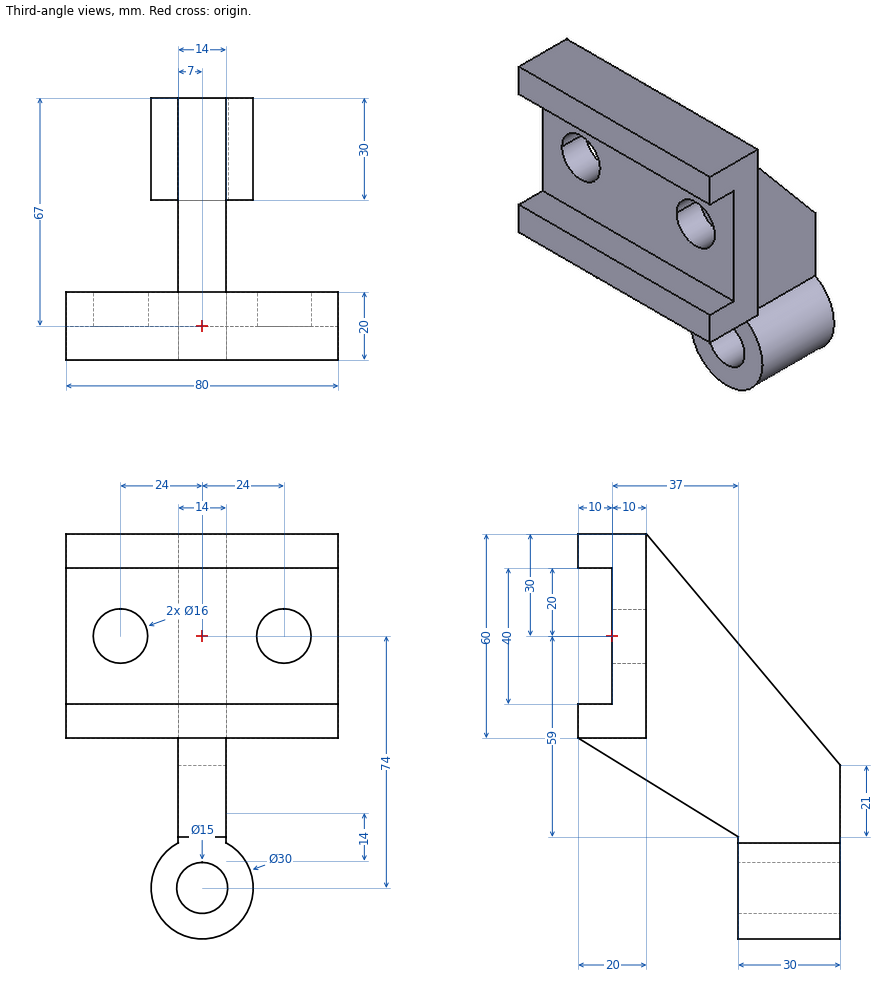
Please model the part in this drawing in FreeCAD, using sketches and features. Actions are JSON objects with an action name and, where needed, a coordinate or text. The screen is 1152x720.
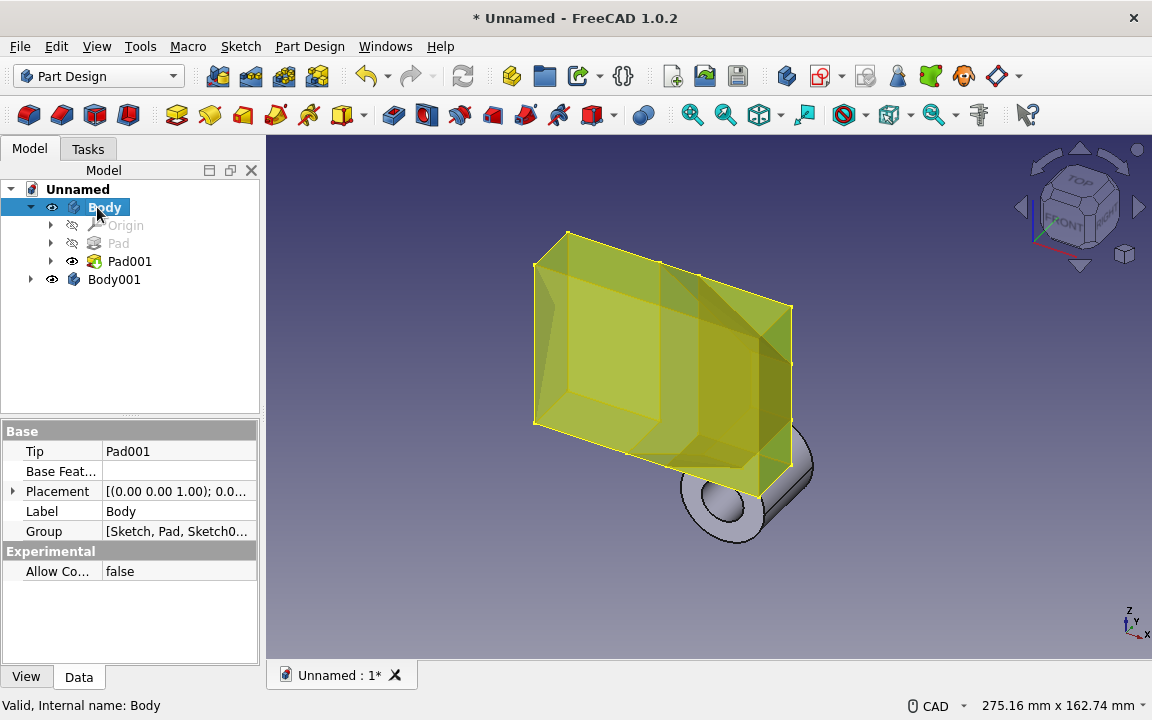
{"action": "left_click", "coordinate": [148, 571]}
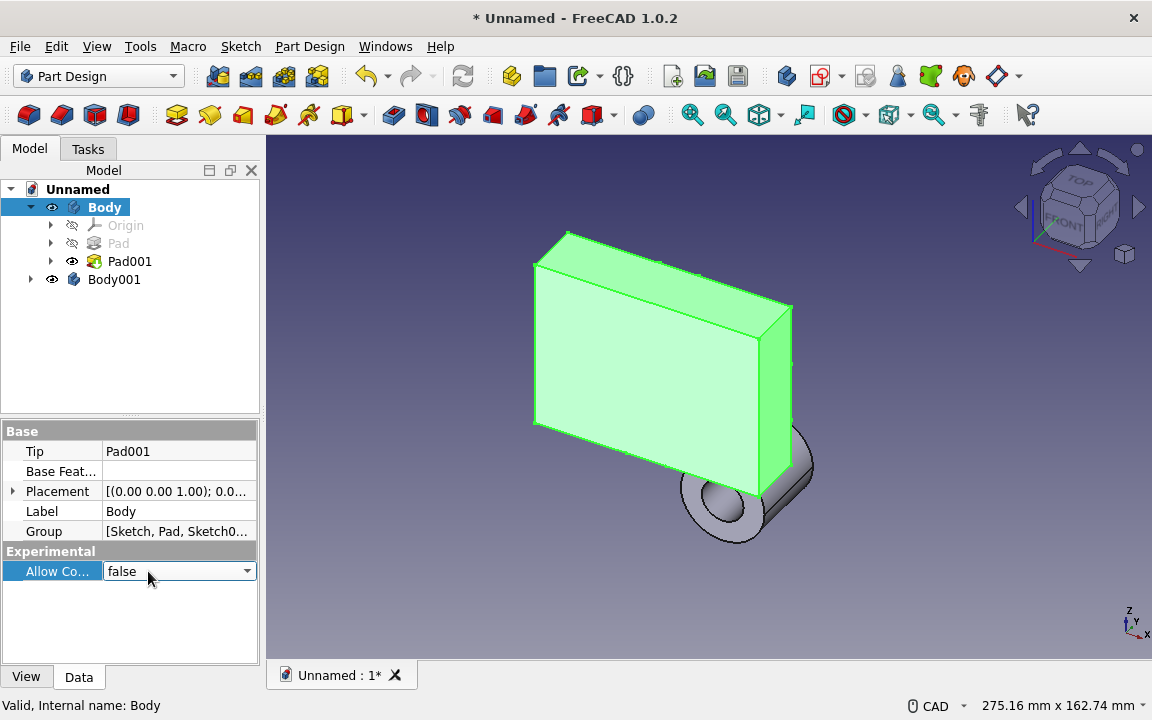
{"action": "left_click", "coordinate": [148, 571]}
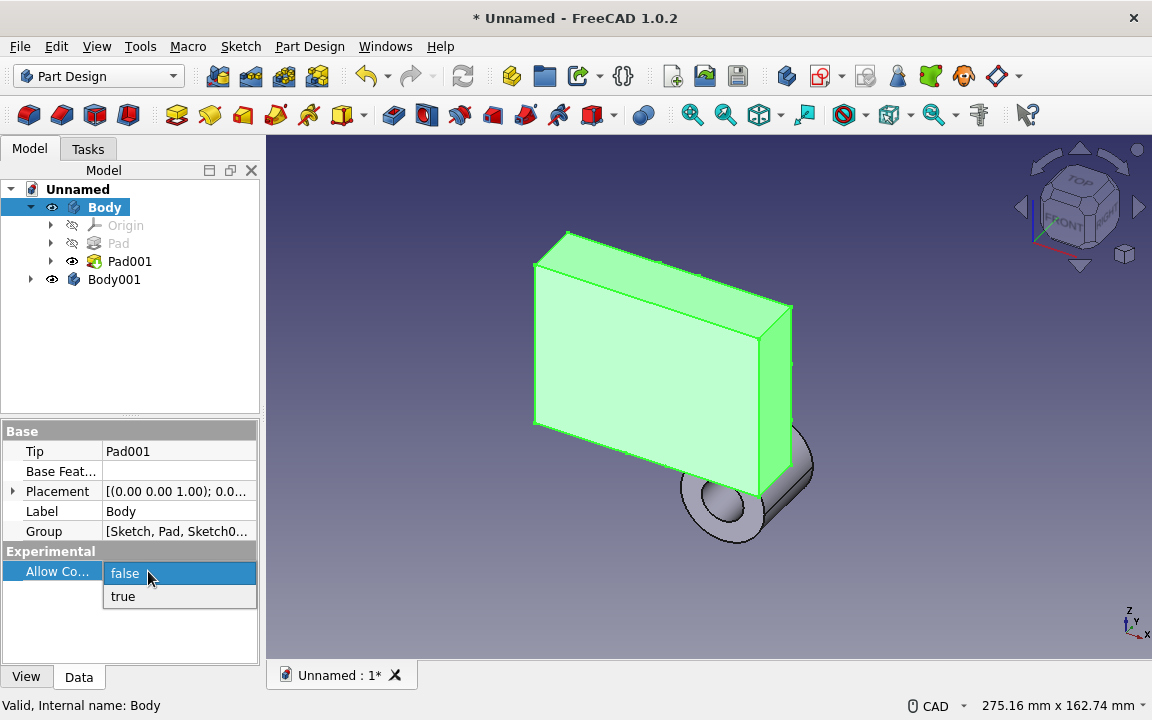
{"action": "left_click", "coordinate": [178, 596]}
{"action": "key", "text": "Return"}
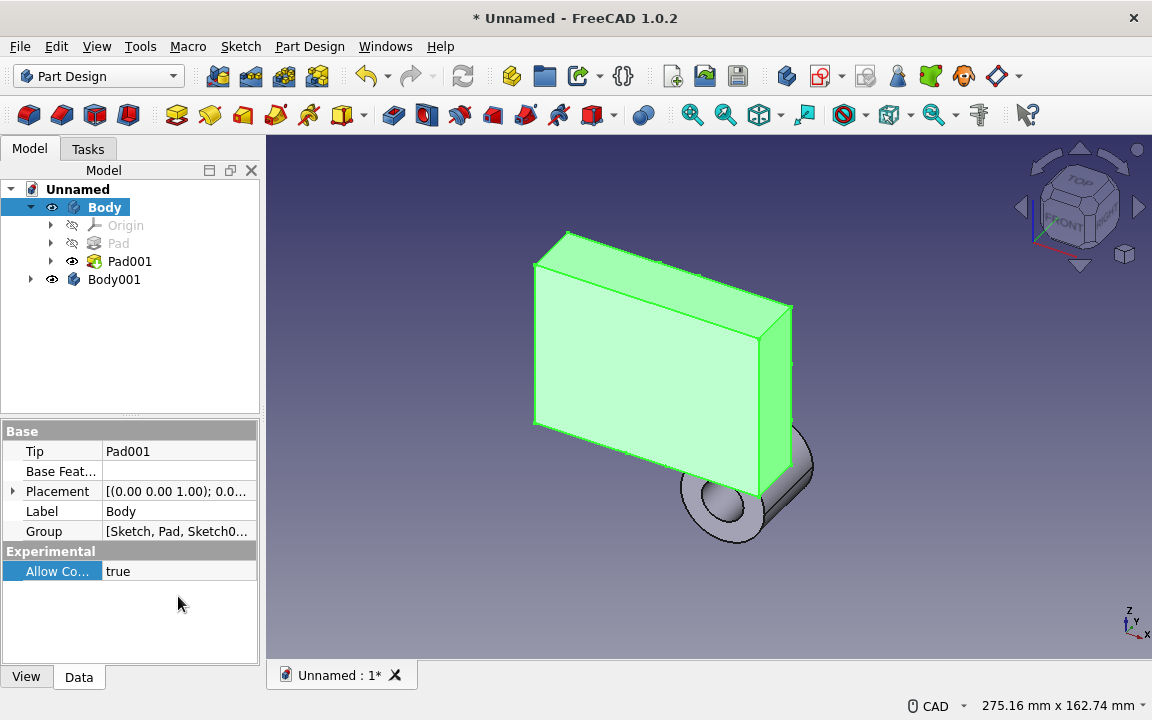
{"action": "left_click", "coordinate": [97, 279]}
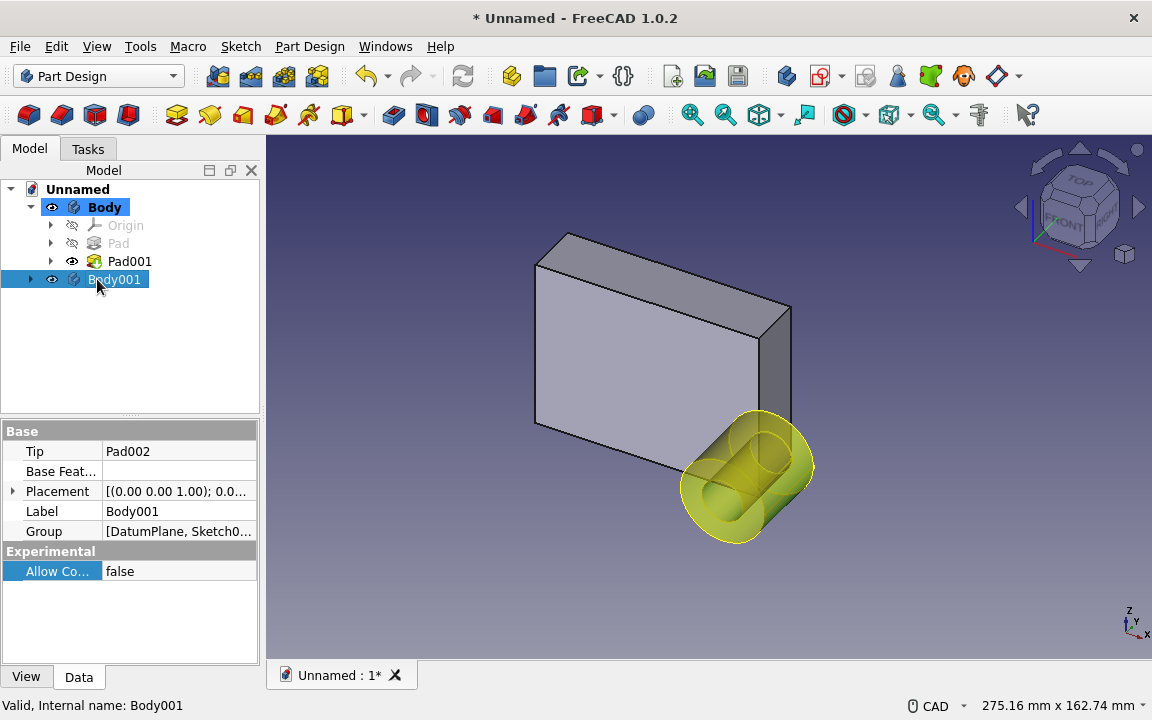
{"action": "left_click", "coordinate": [644, 116]}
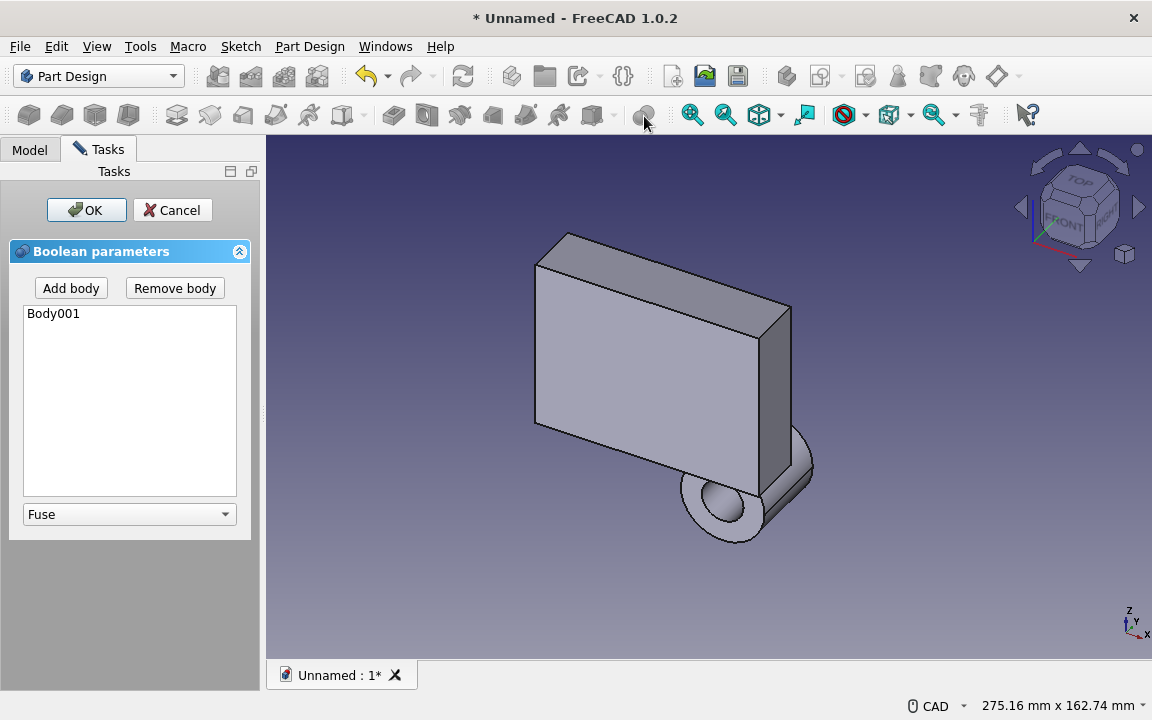
{"action": "left_click", "coordinate": [87, 210]}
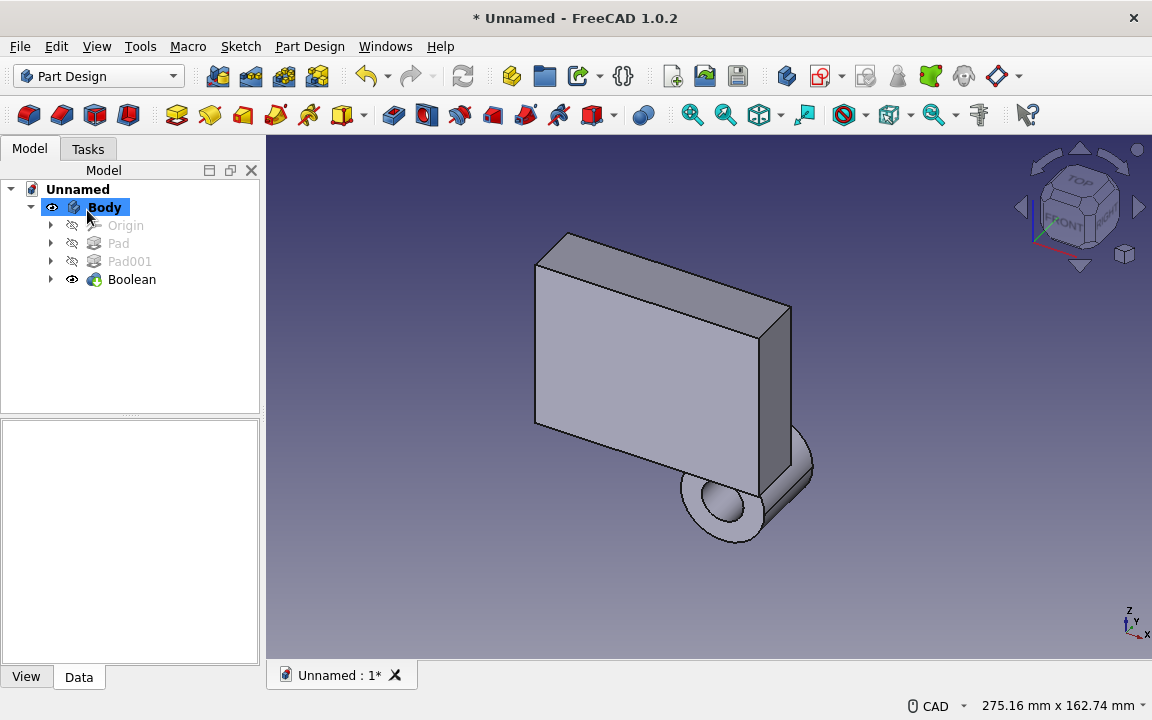
{"action": "left_click", "coordinate": [51, 225]}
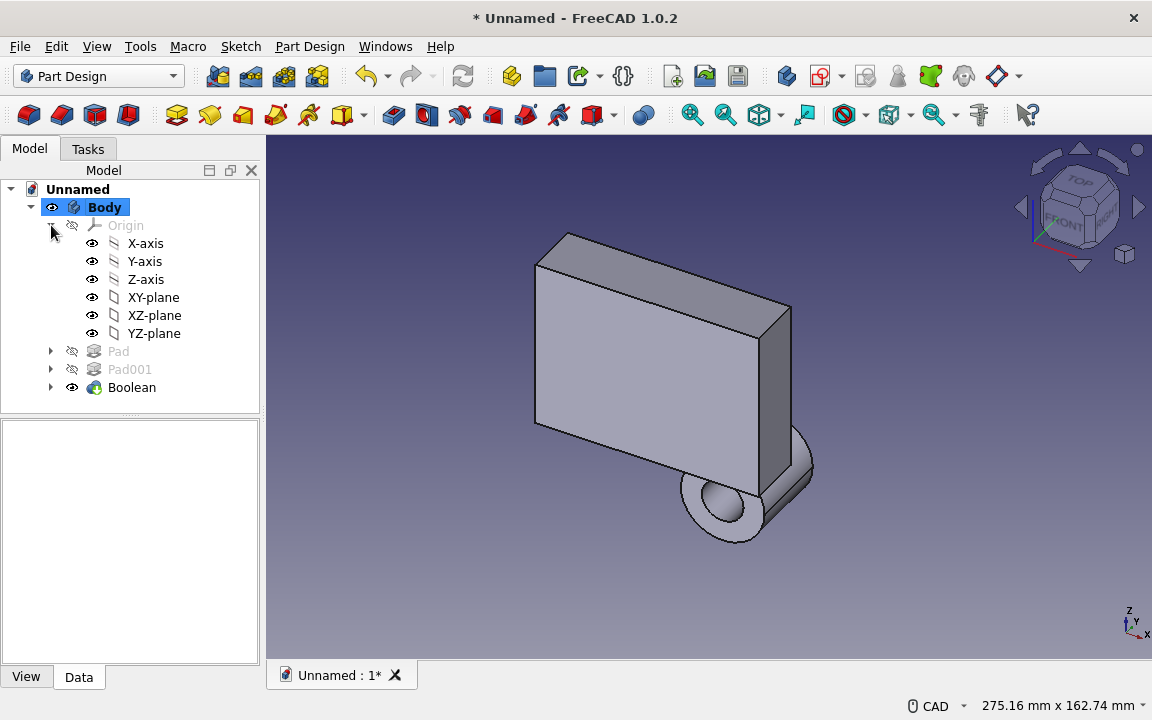
{"action": "left_click", "coordinate": [137, 297]}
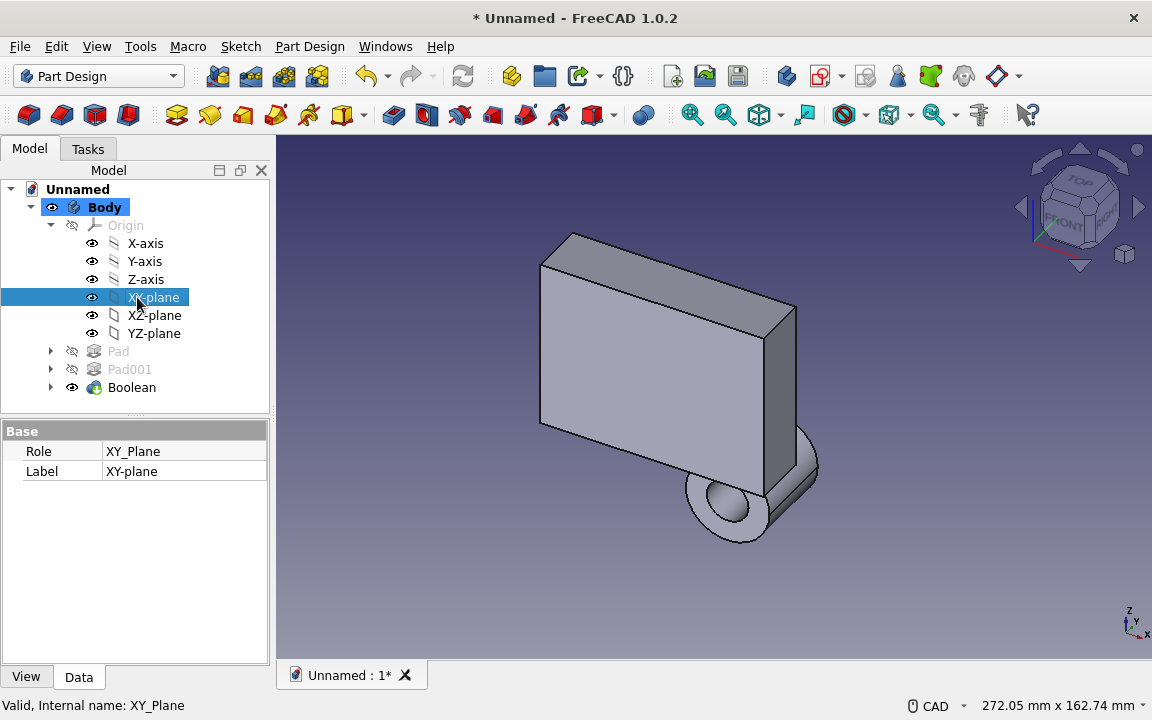
{"action": "left_click", "coordinate": [996, 76]}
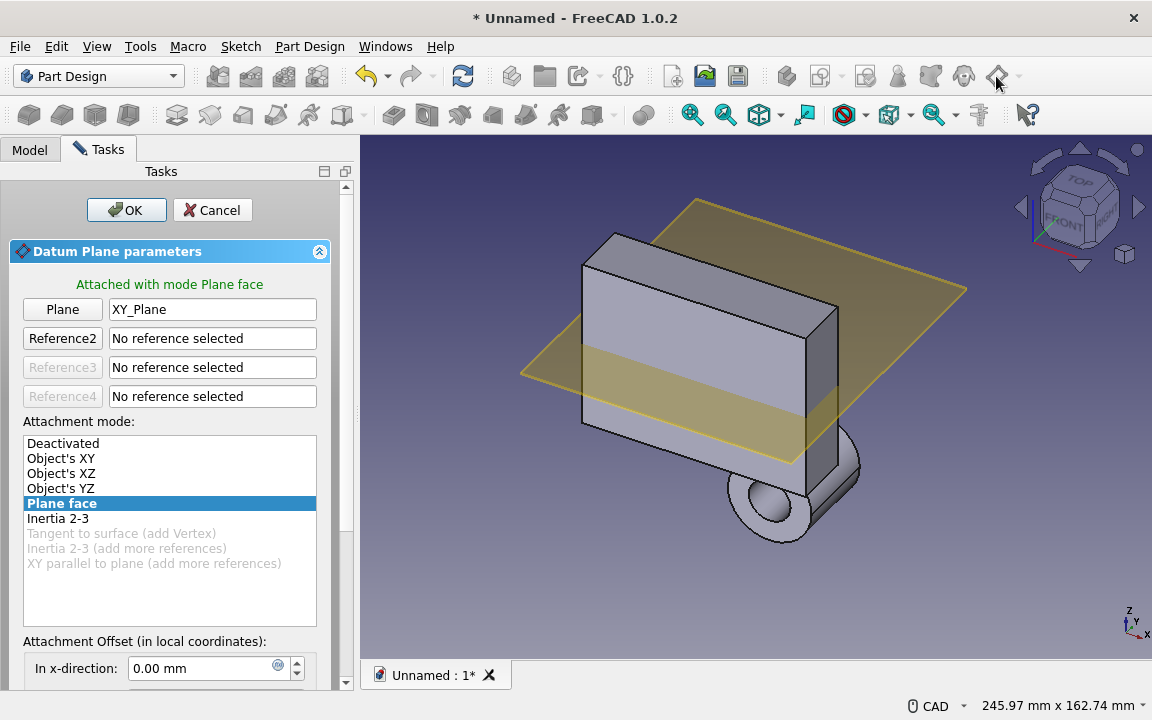
{"action": "scroll", "coordinate": [346, 436], "scroll_direction": "down", "scroll_amount": 2}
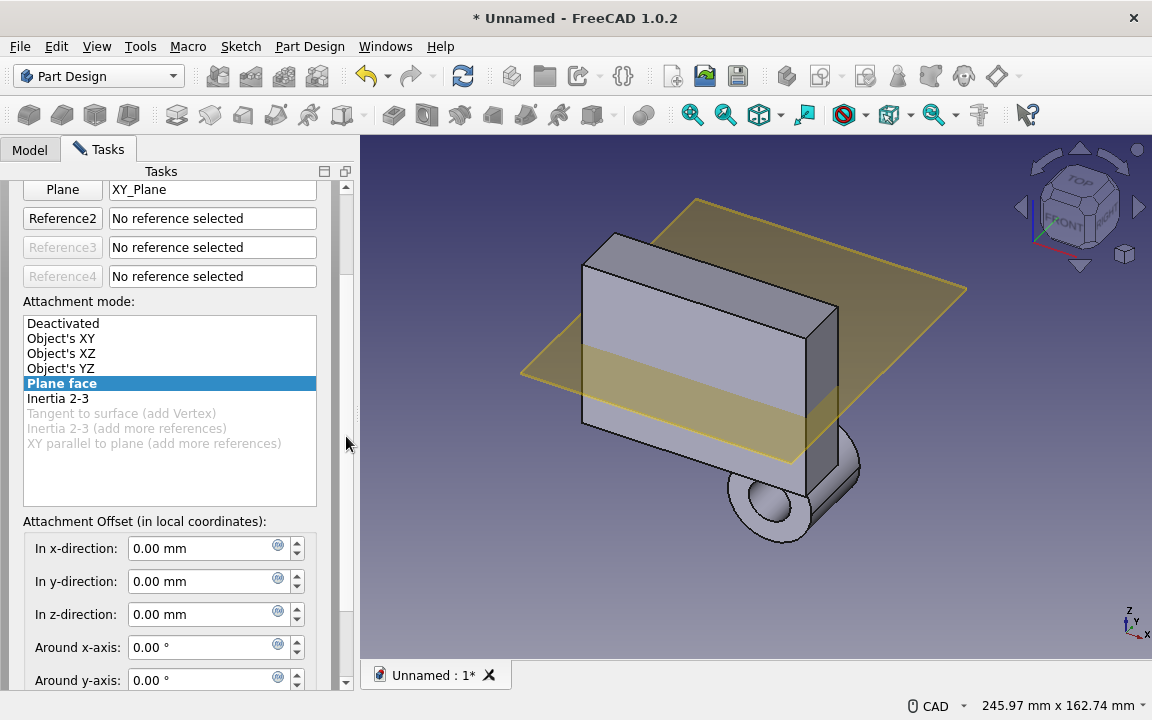
{"action": "triple_click", "coordinate": [210, 614]}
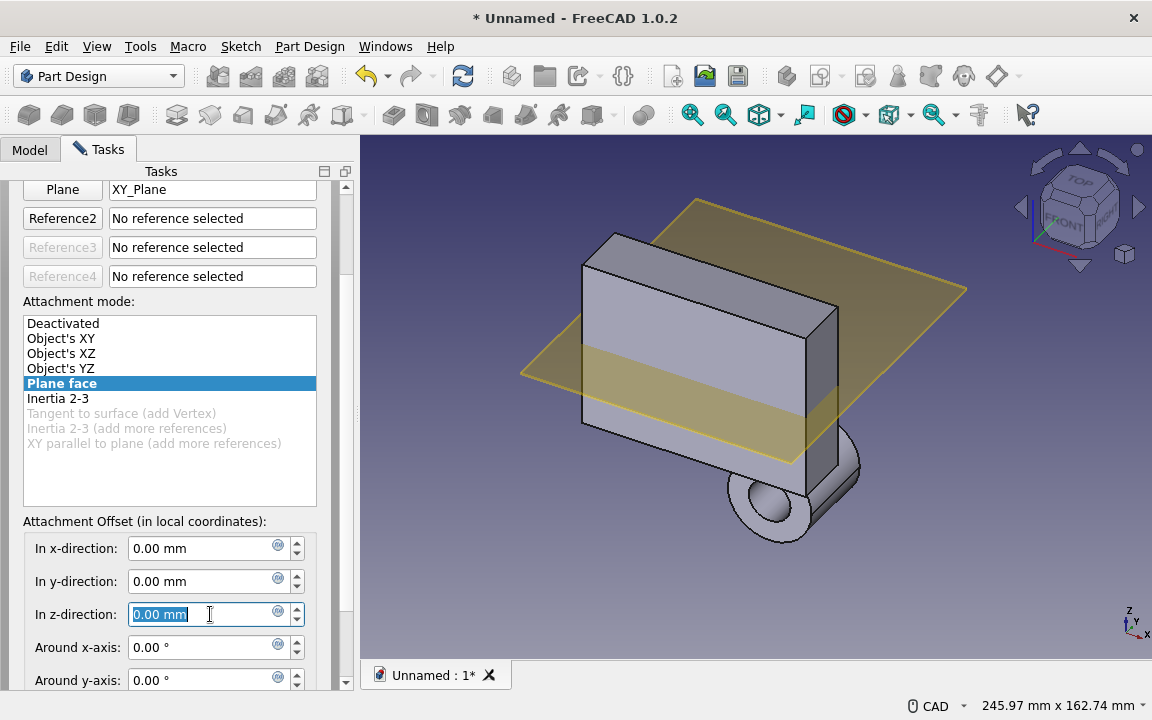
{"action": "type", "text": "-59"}
{"action": "key", "text": "Tab"}